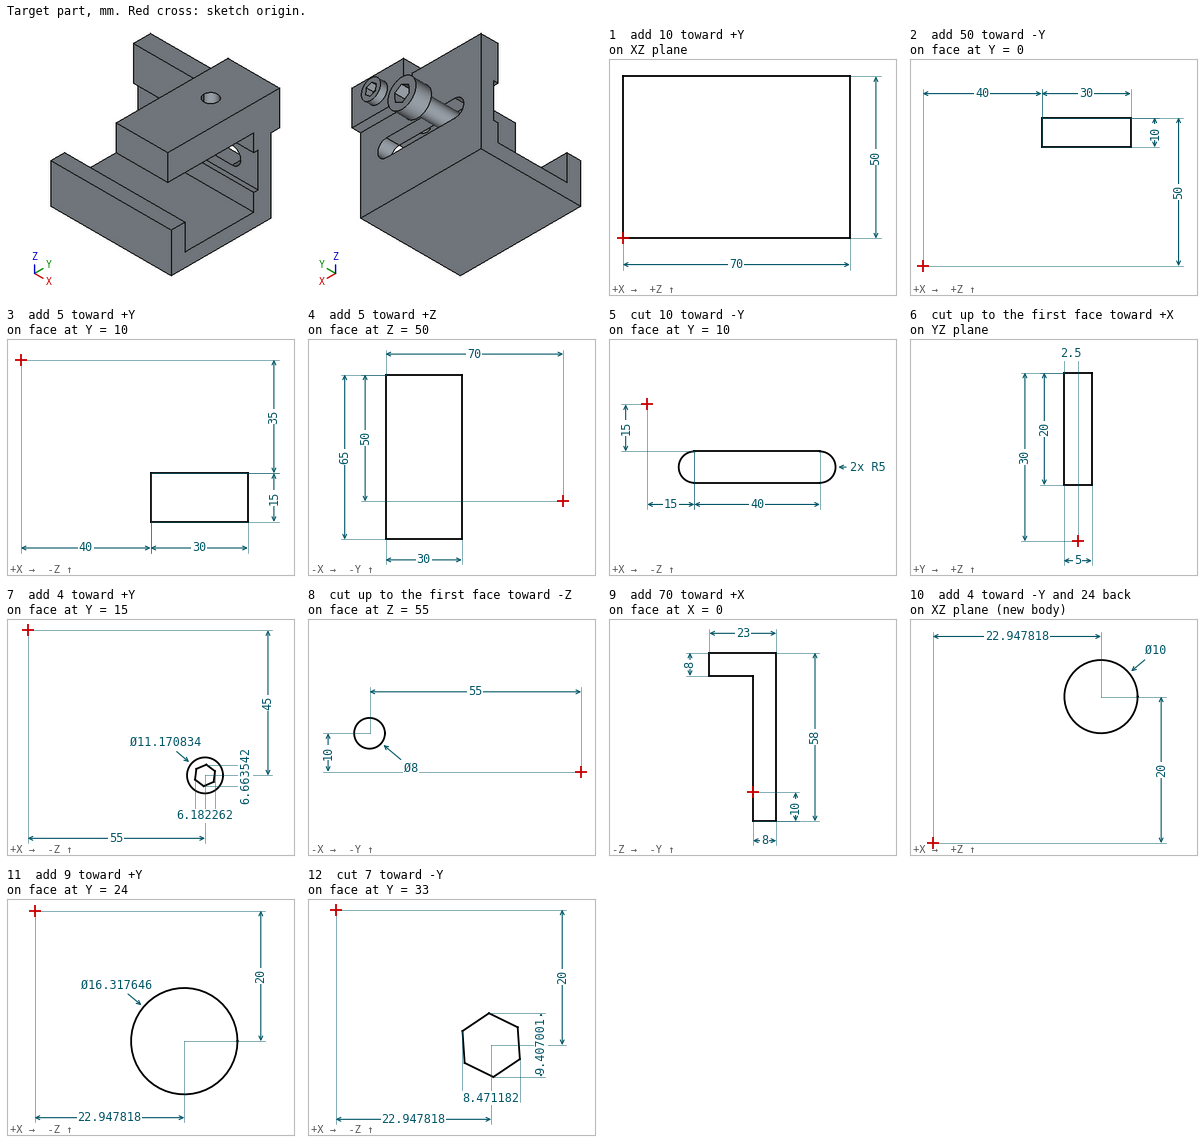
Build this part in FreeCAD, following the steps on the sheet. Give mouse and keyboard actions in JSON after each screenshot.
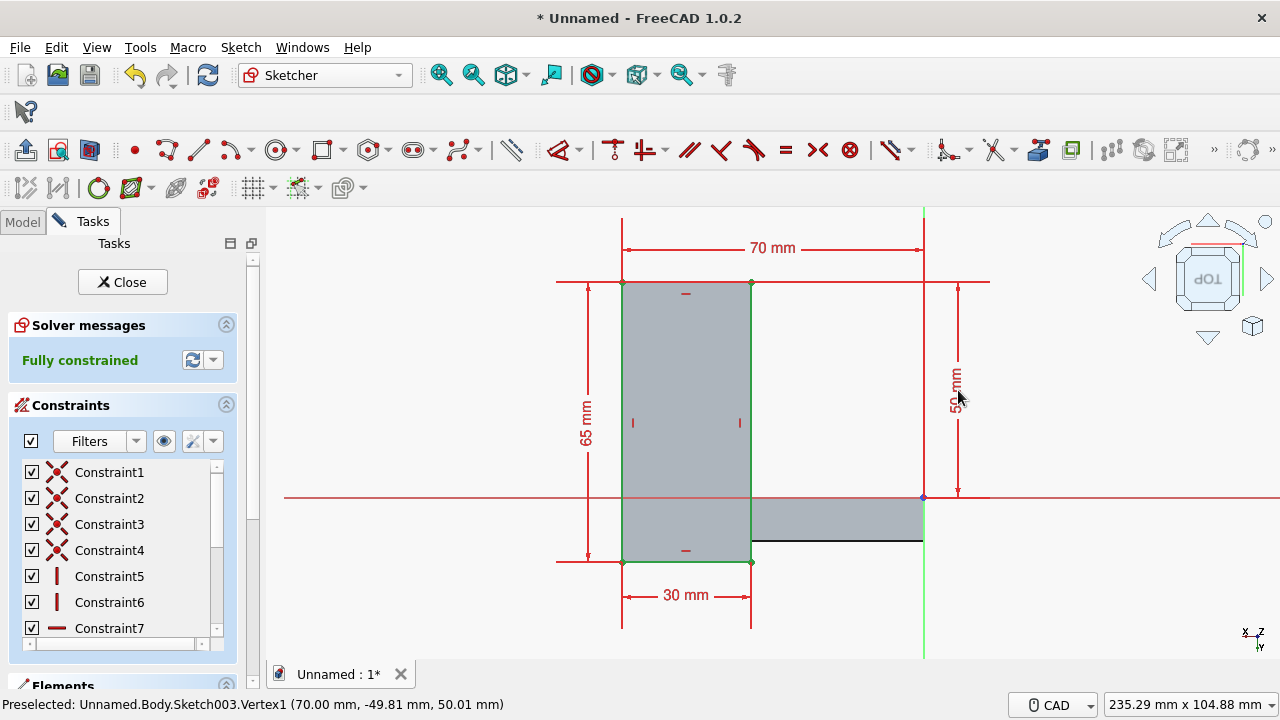
{"action": "left_click", "coordinate": [123, 282]}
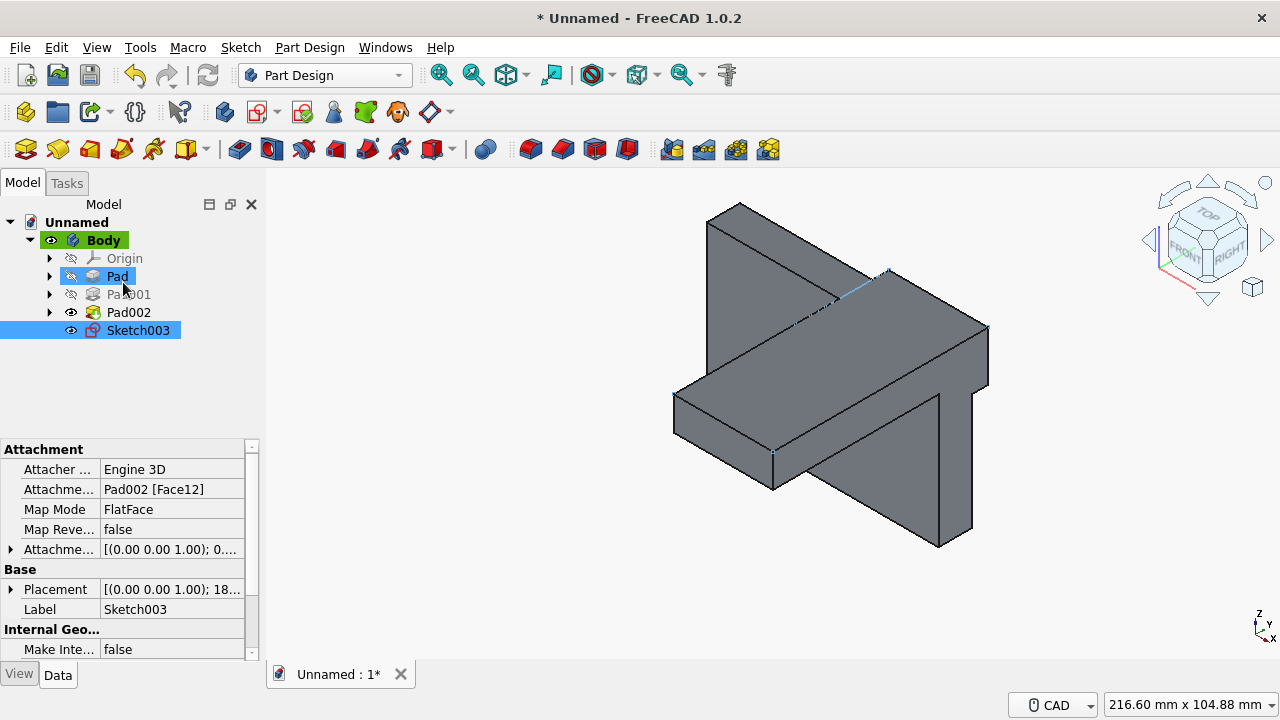
{"action": "left_click", "coordinate": [26, 150]}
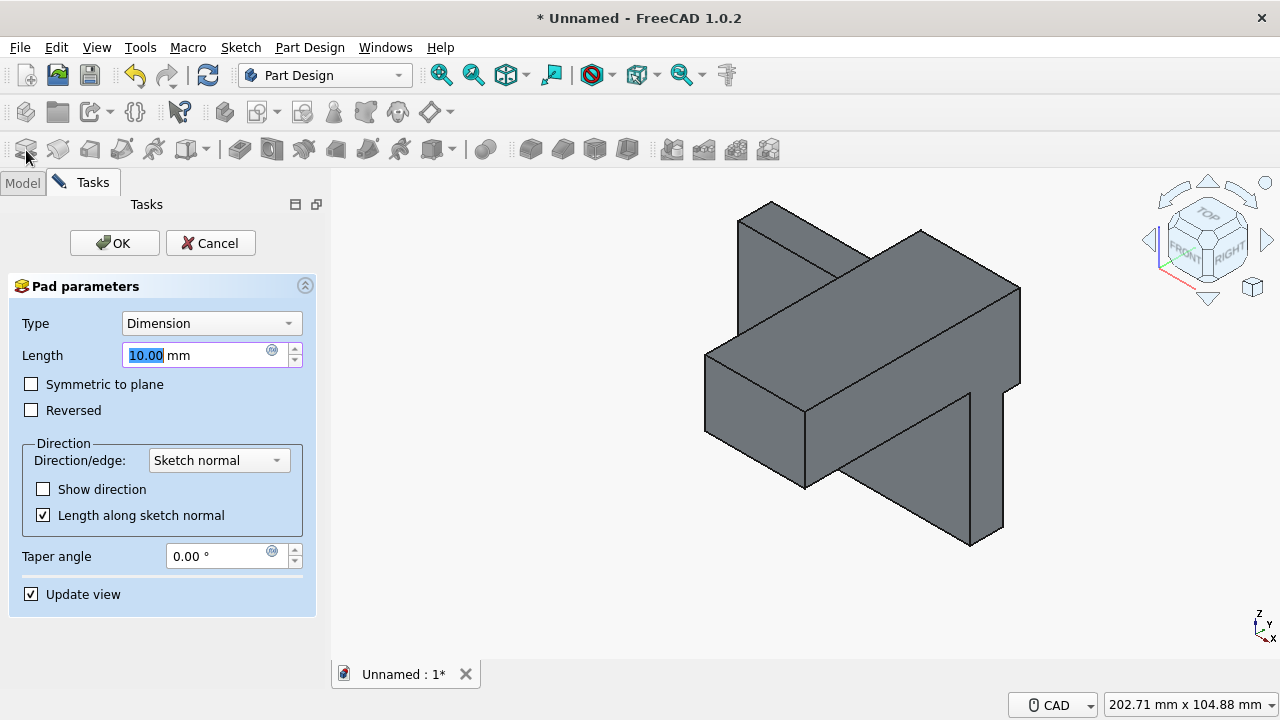
{"action": "type", "text": "5"}
{"action": "key", "text": "Tab"}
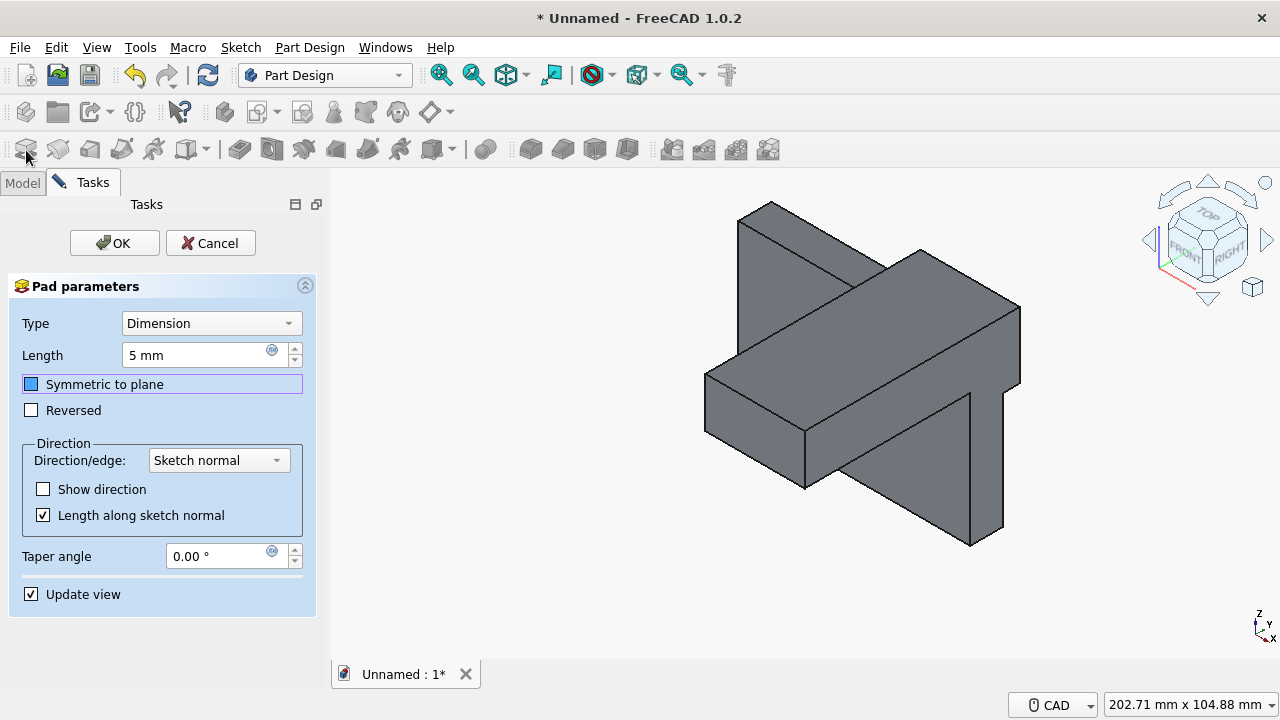
{"action": "left_click", "coordinate": [115, 243]}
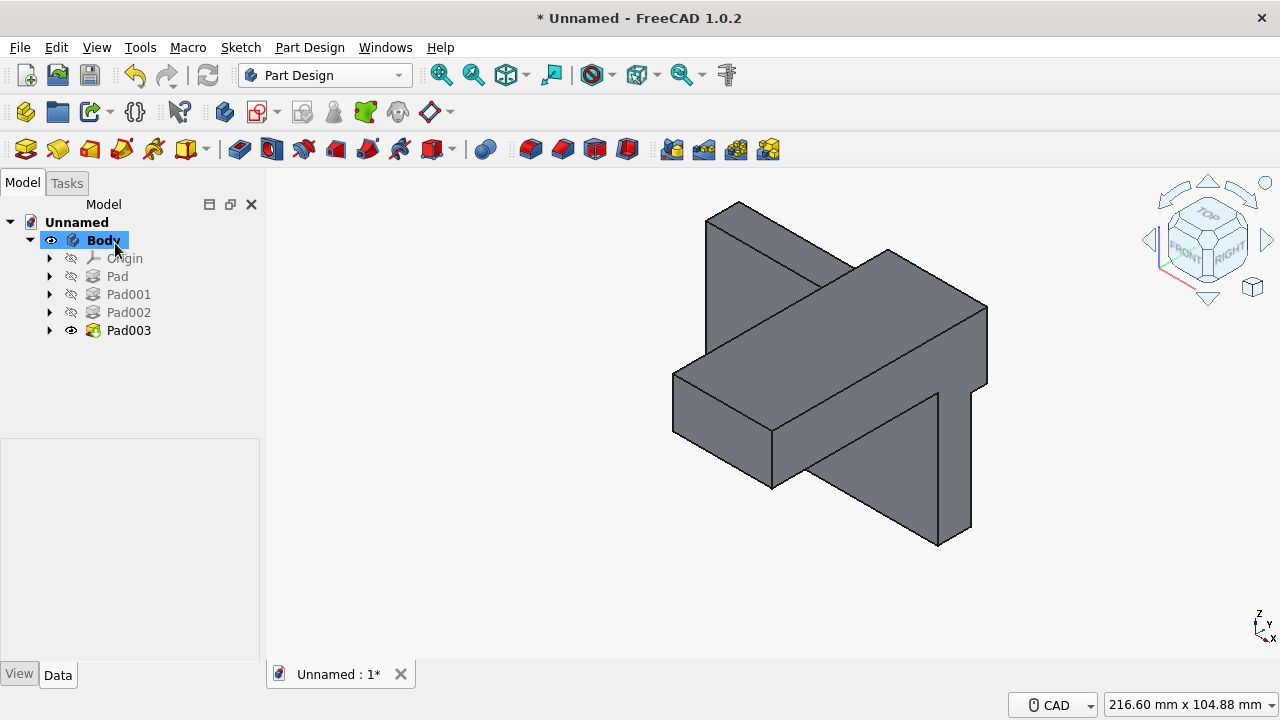
{"action": "key", "text": "4"}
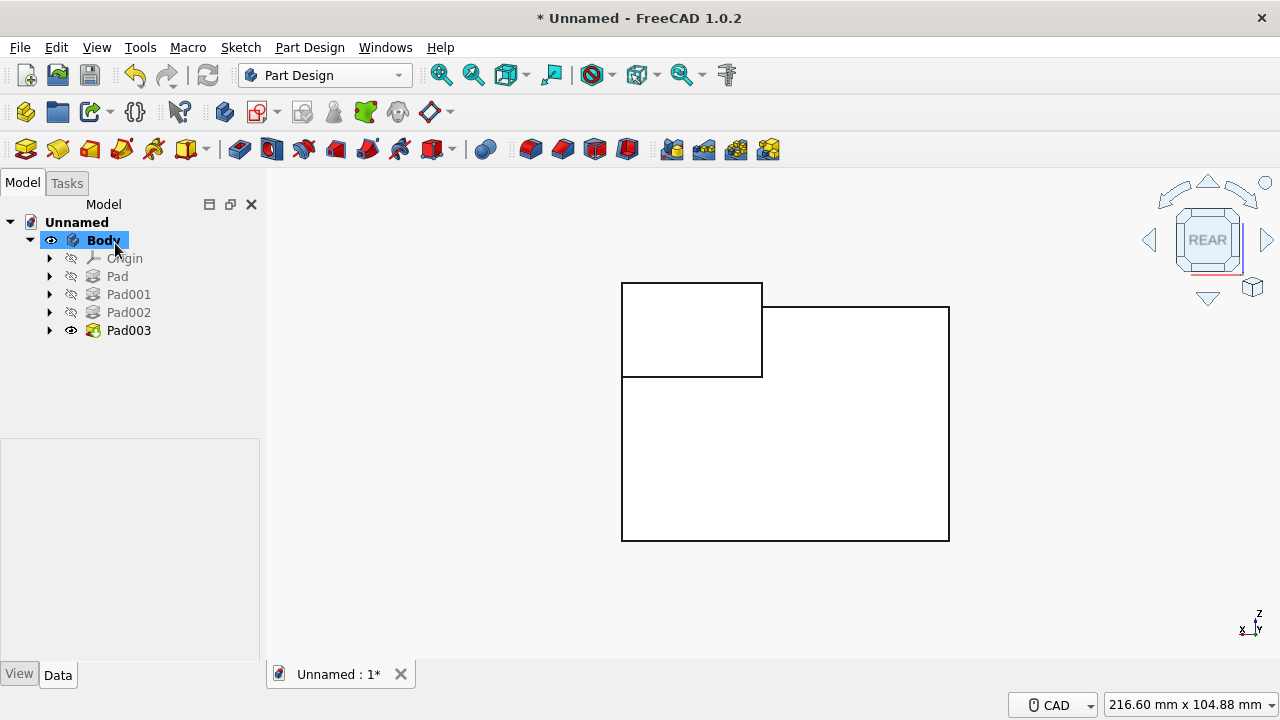
{"action": "left_click", "coordinate": [832, 423]}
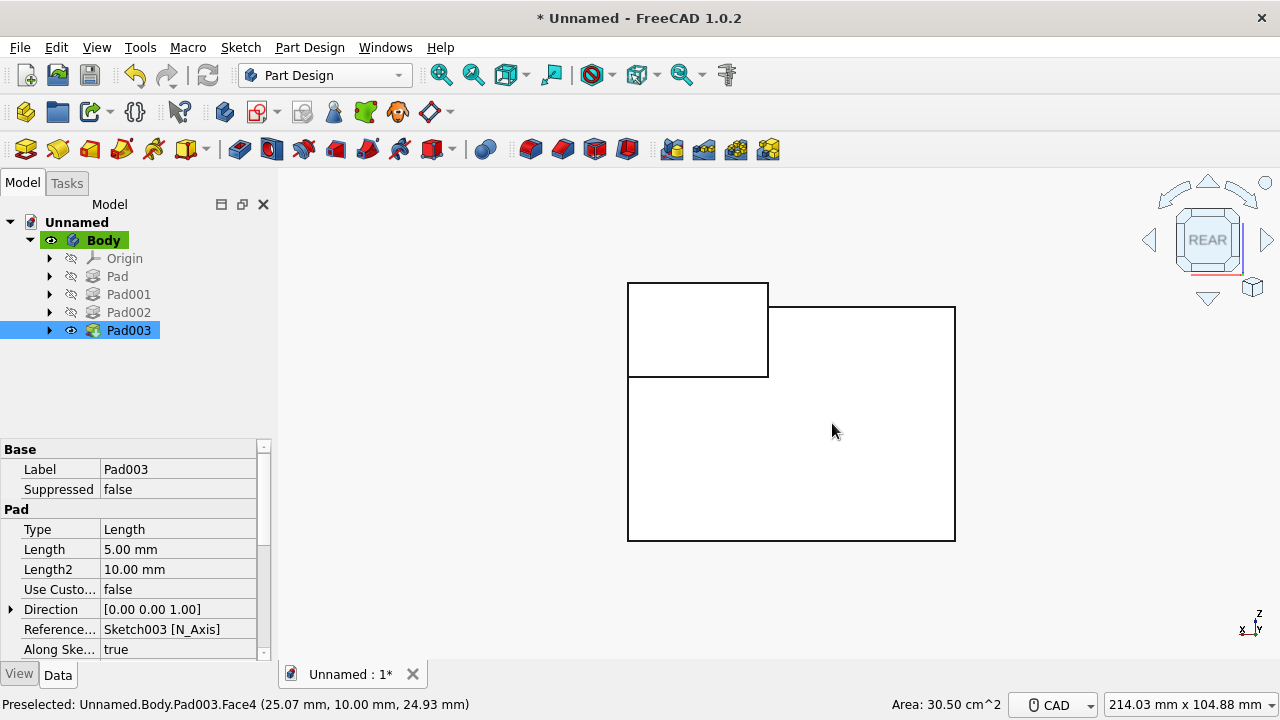
{"action": "left_click", "coordinate": [258, 112]}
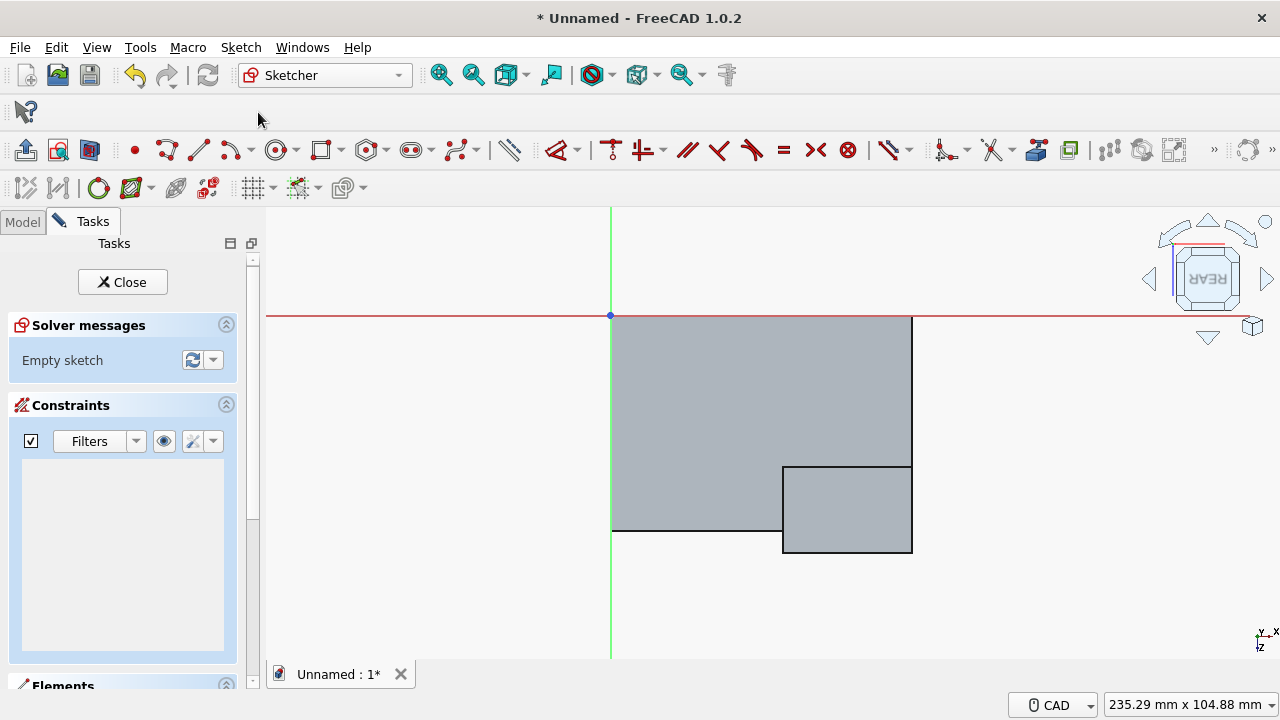
{"action": "scroll", "coordinate": [769, 318], "scroll_direction": "up", "scroll_amount": 4}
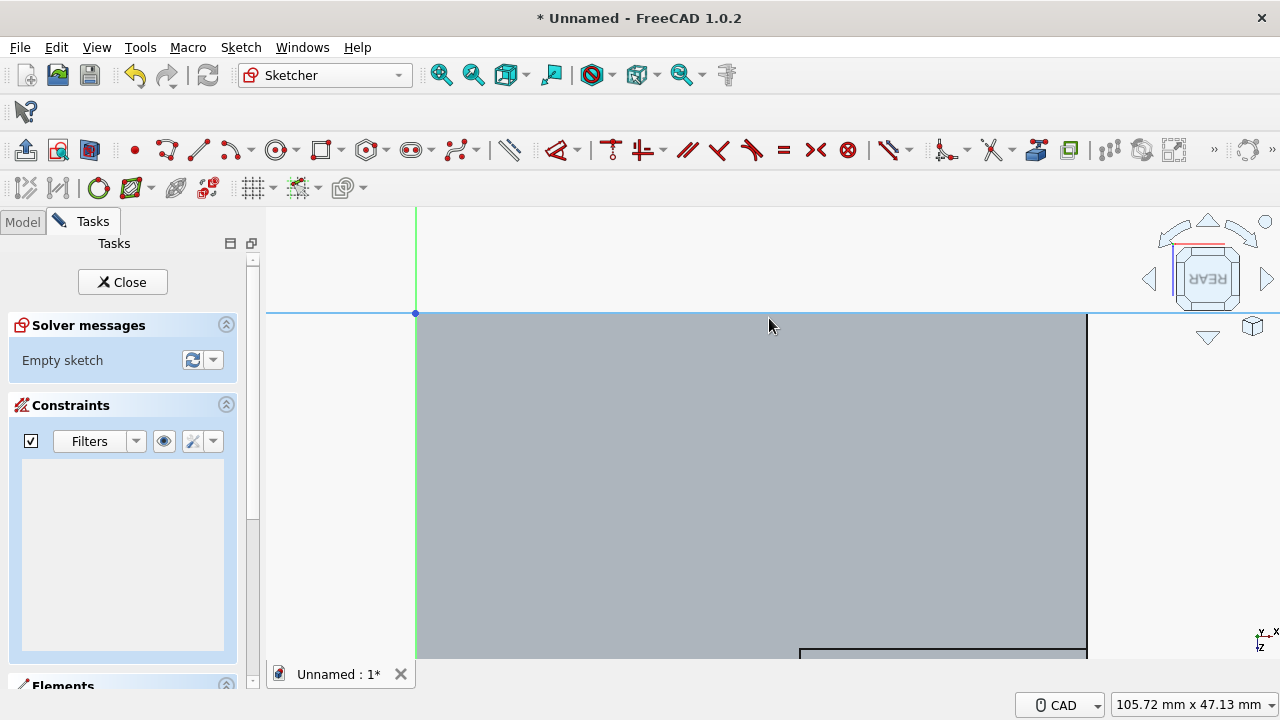
{"action": "left_click", "coordinate": [412, 150]}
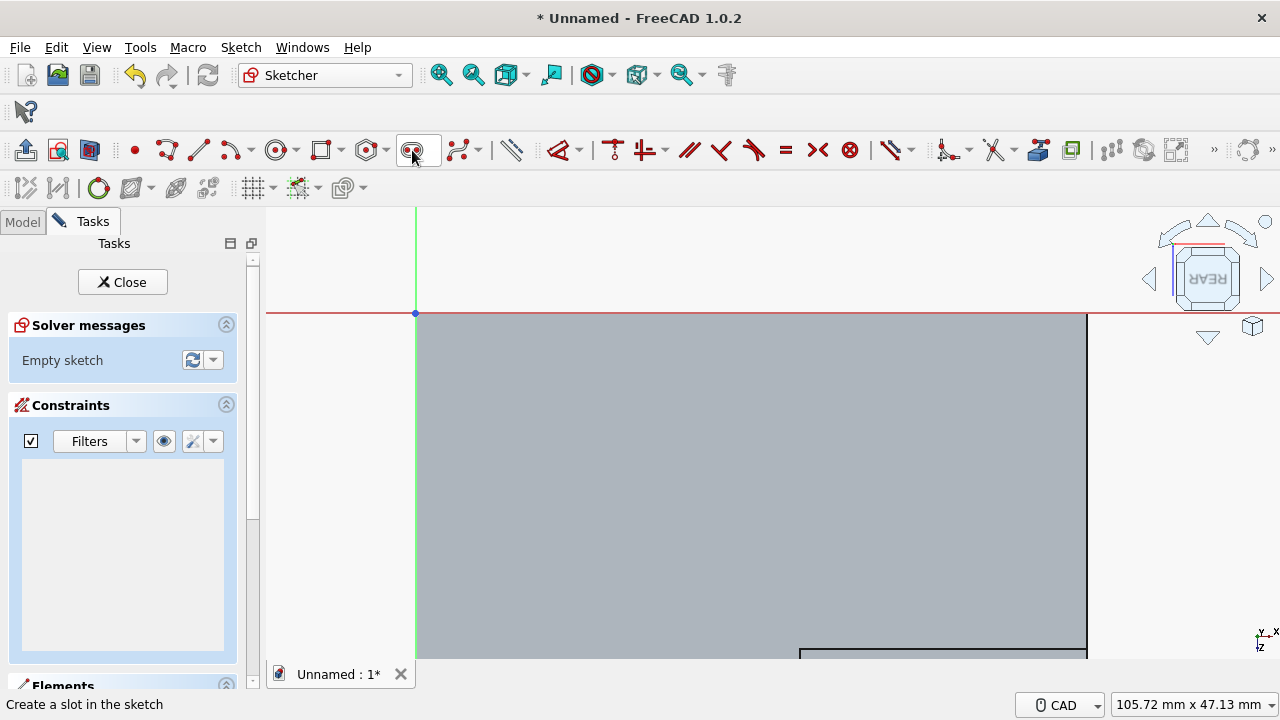
{"action": "left_click", "coordinate": [560, 505]}